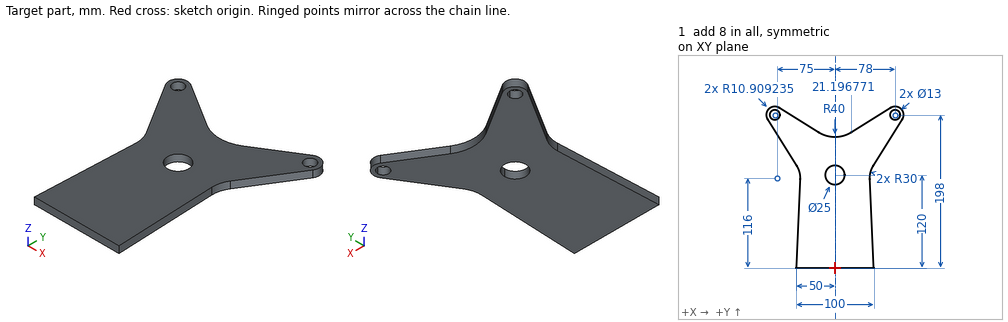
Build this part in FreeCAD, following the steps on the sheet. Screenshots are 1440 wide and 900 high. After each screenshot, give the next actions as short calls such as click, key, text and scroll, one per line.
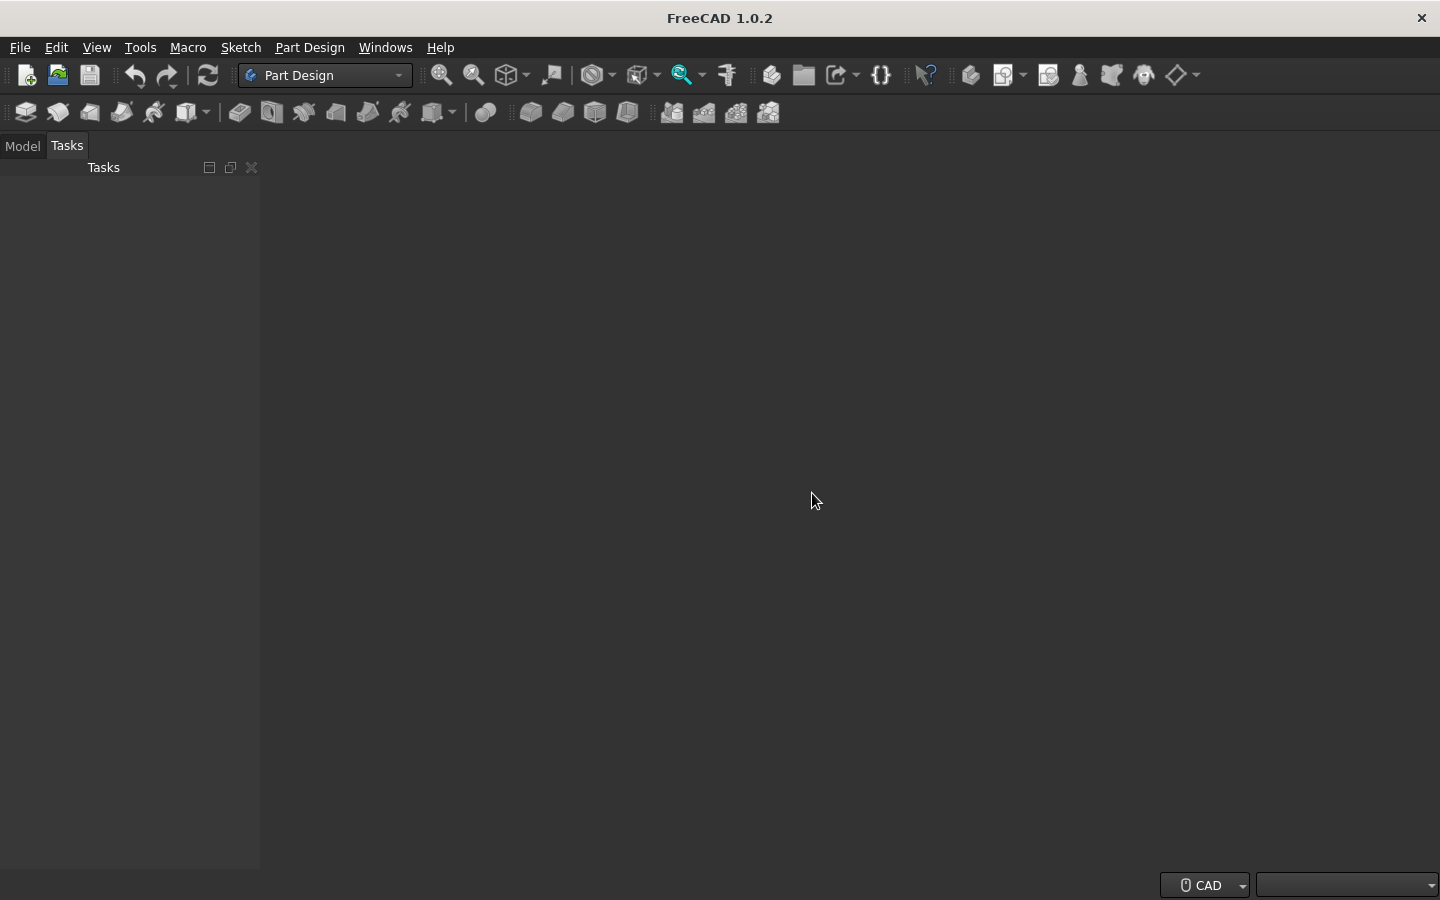
click(26, 76)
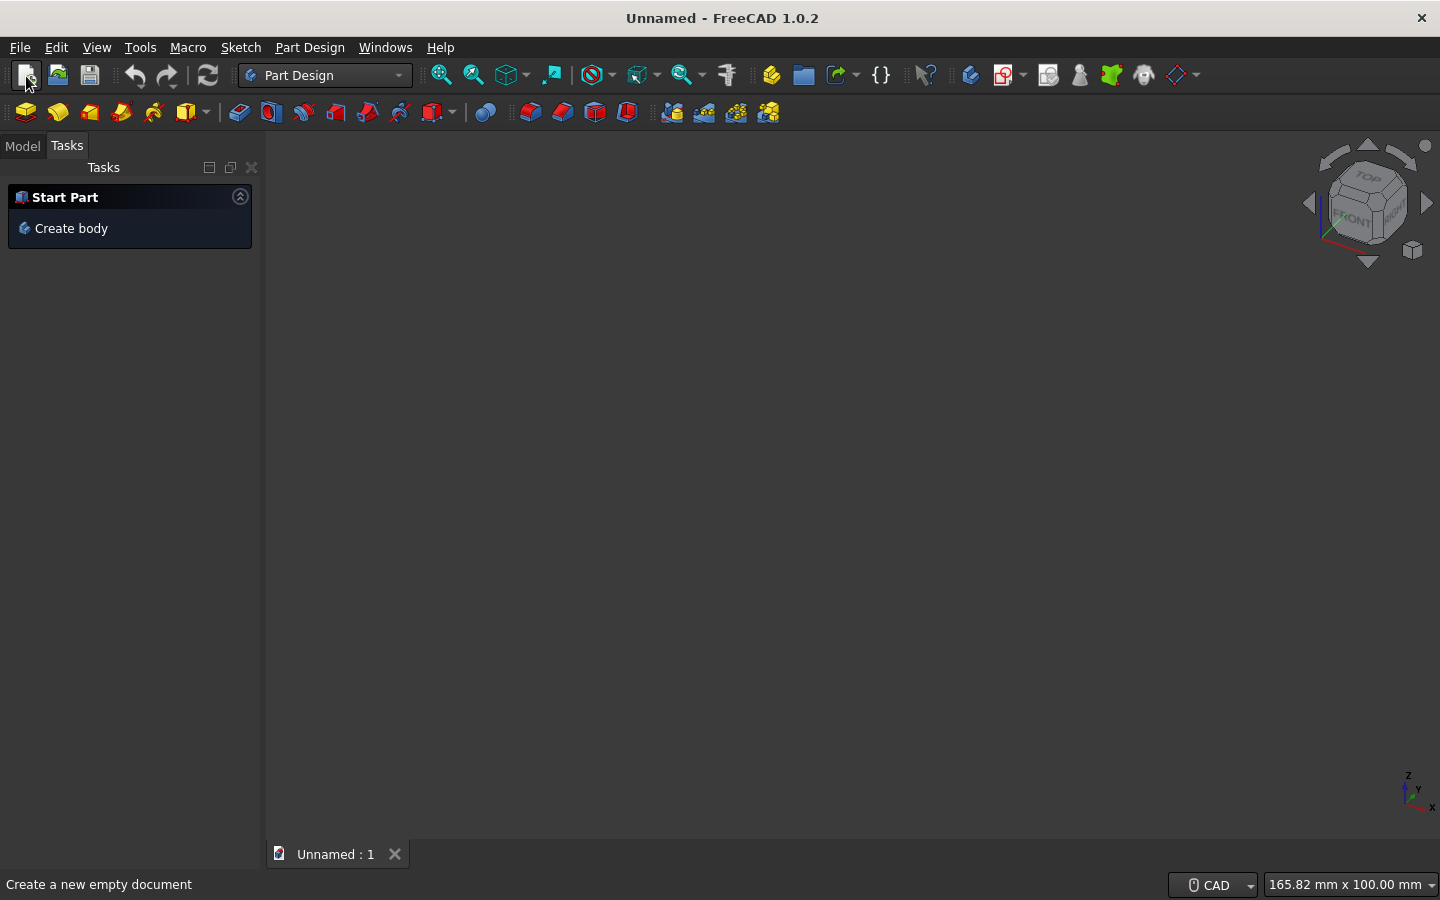
click(1004, 76)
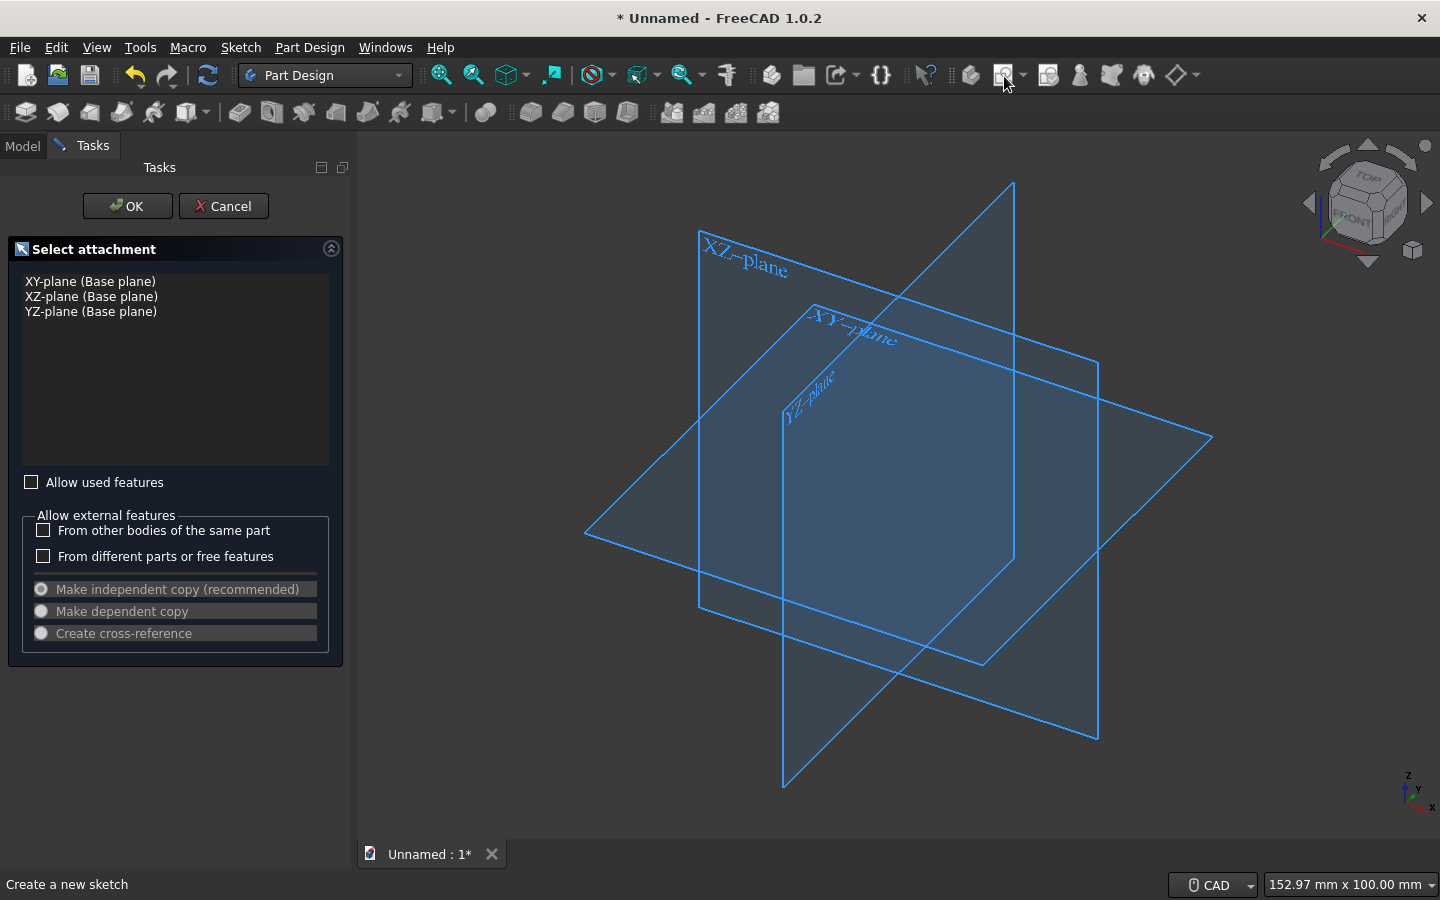
click(82, 282)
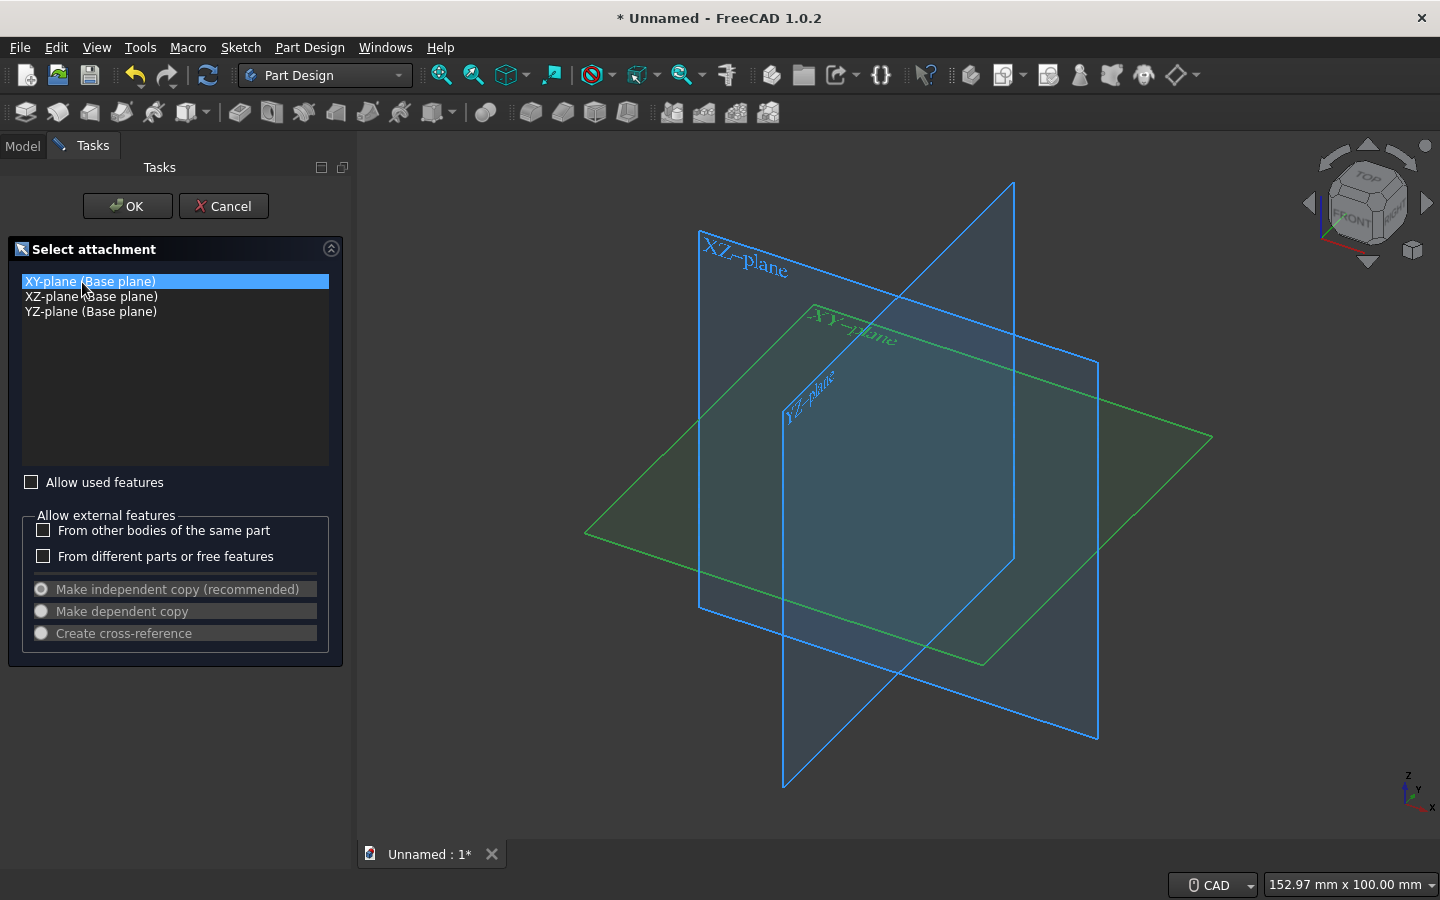
click(128, 206)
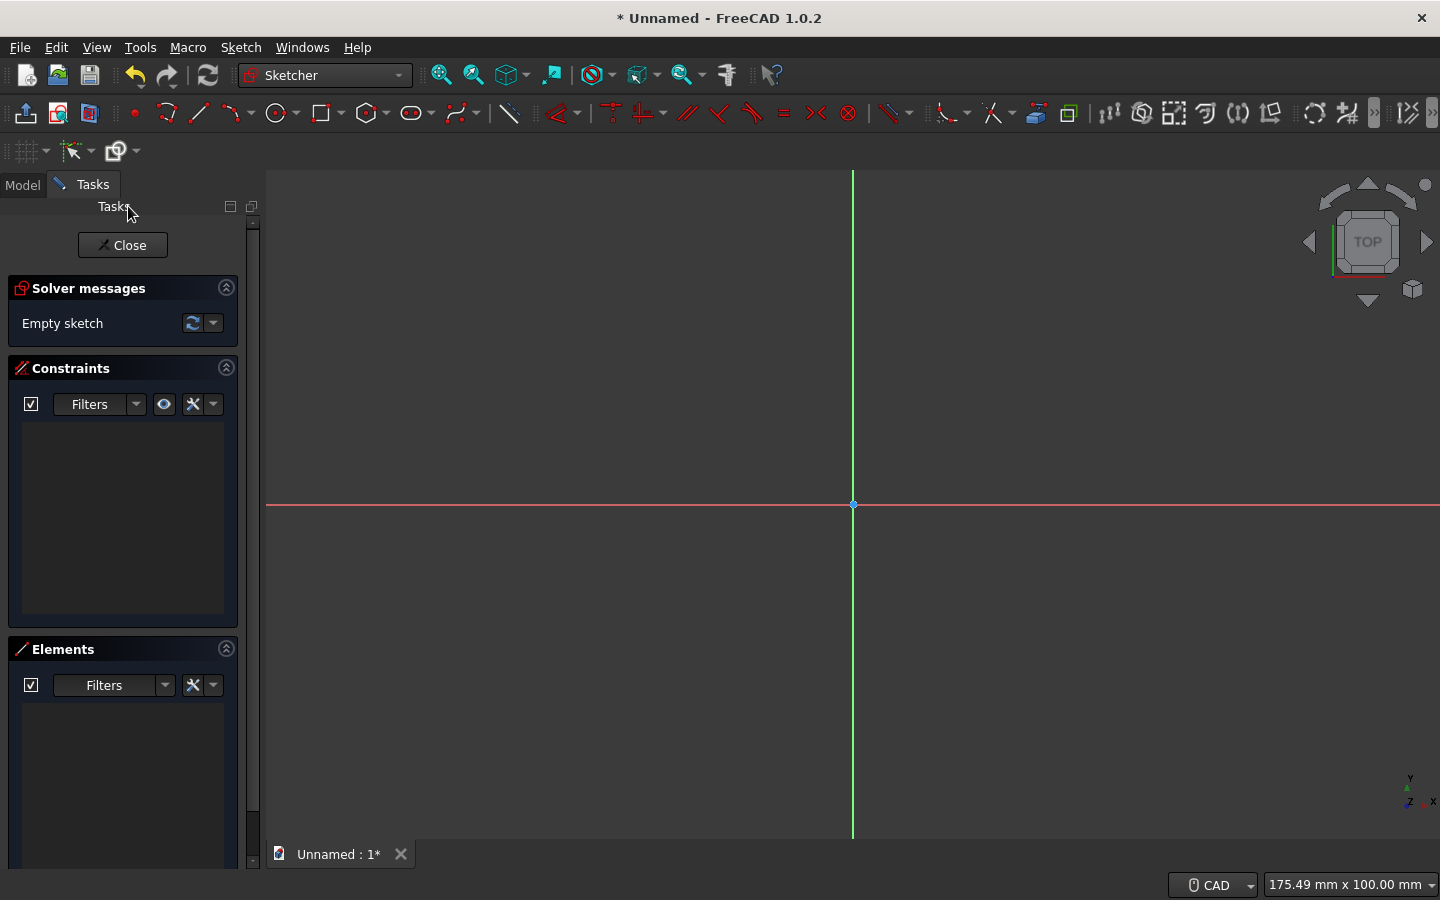
scroll(755, 803, down, 6)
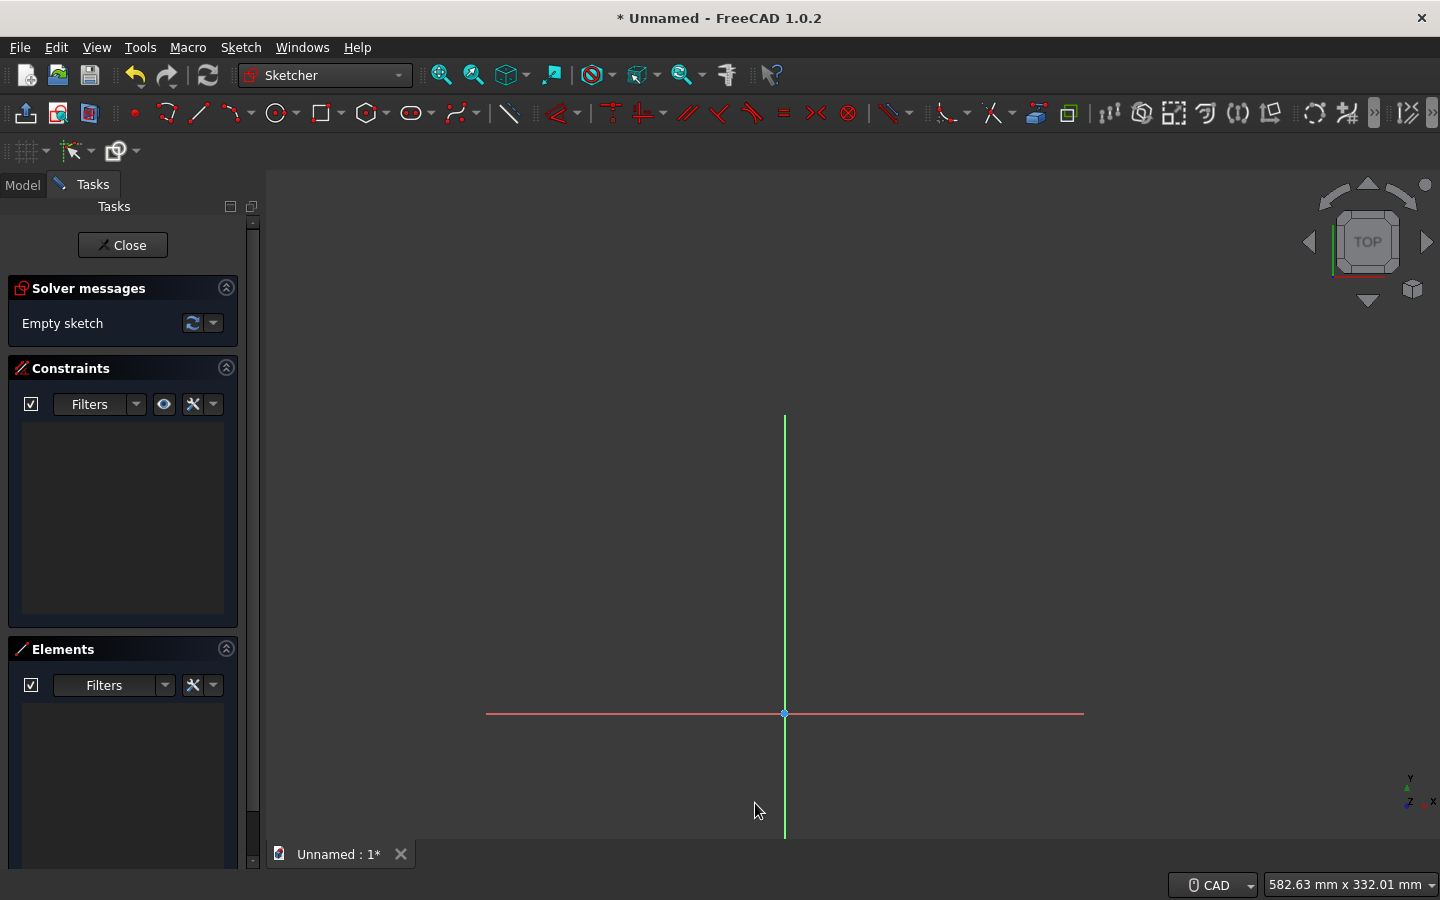
click(200, 114)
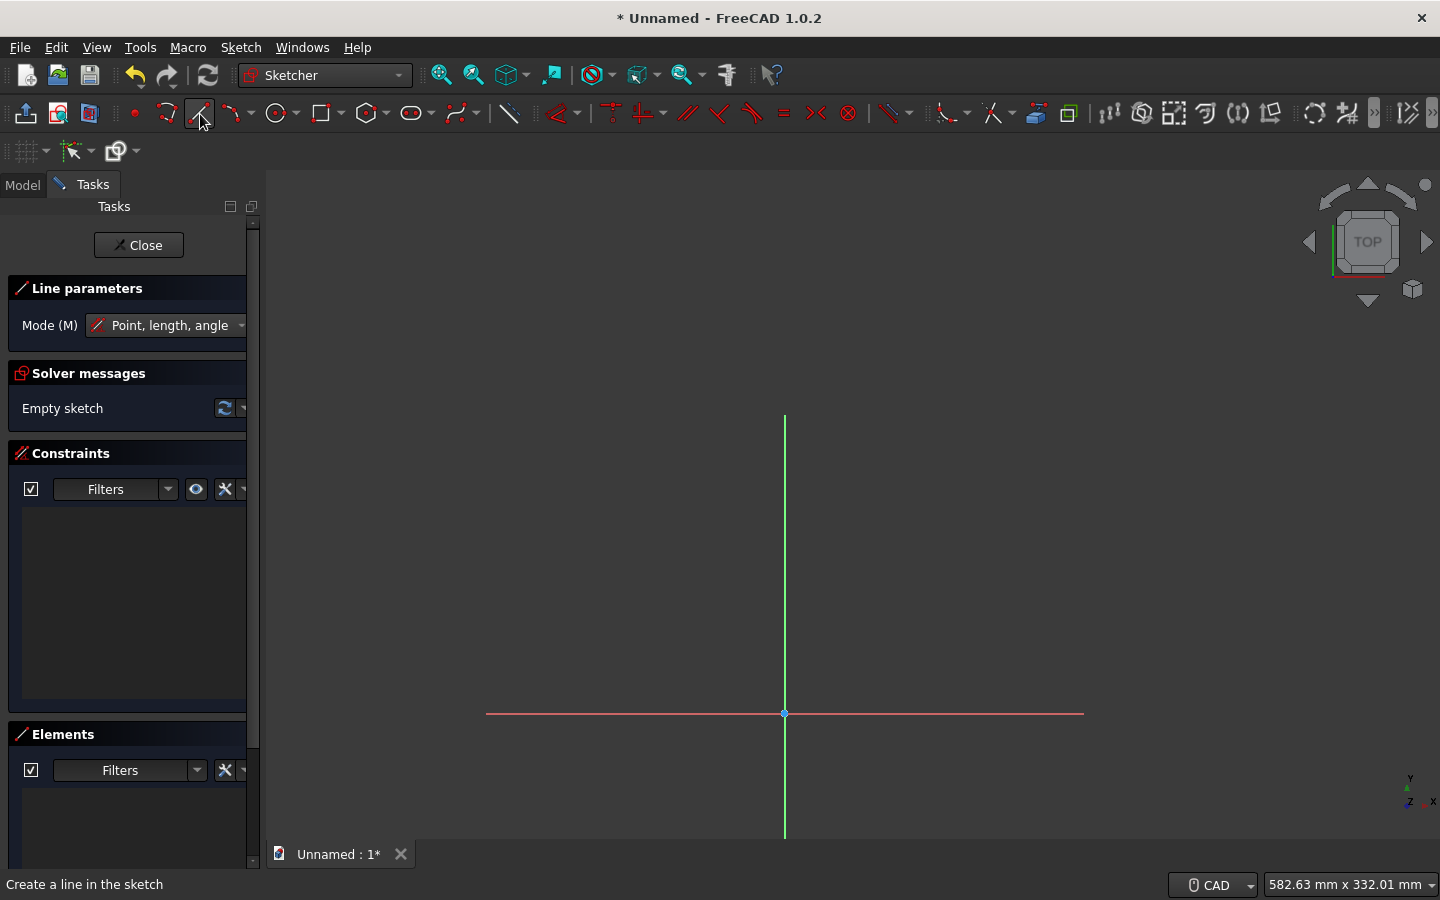
click(885, 448)
click(961, 326)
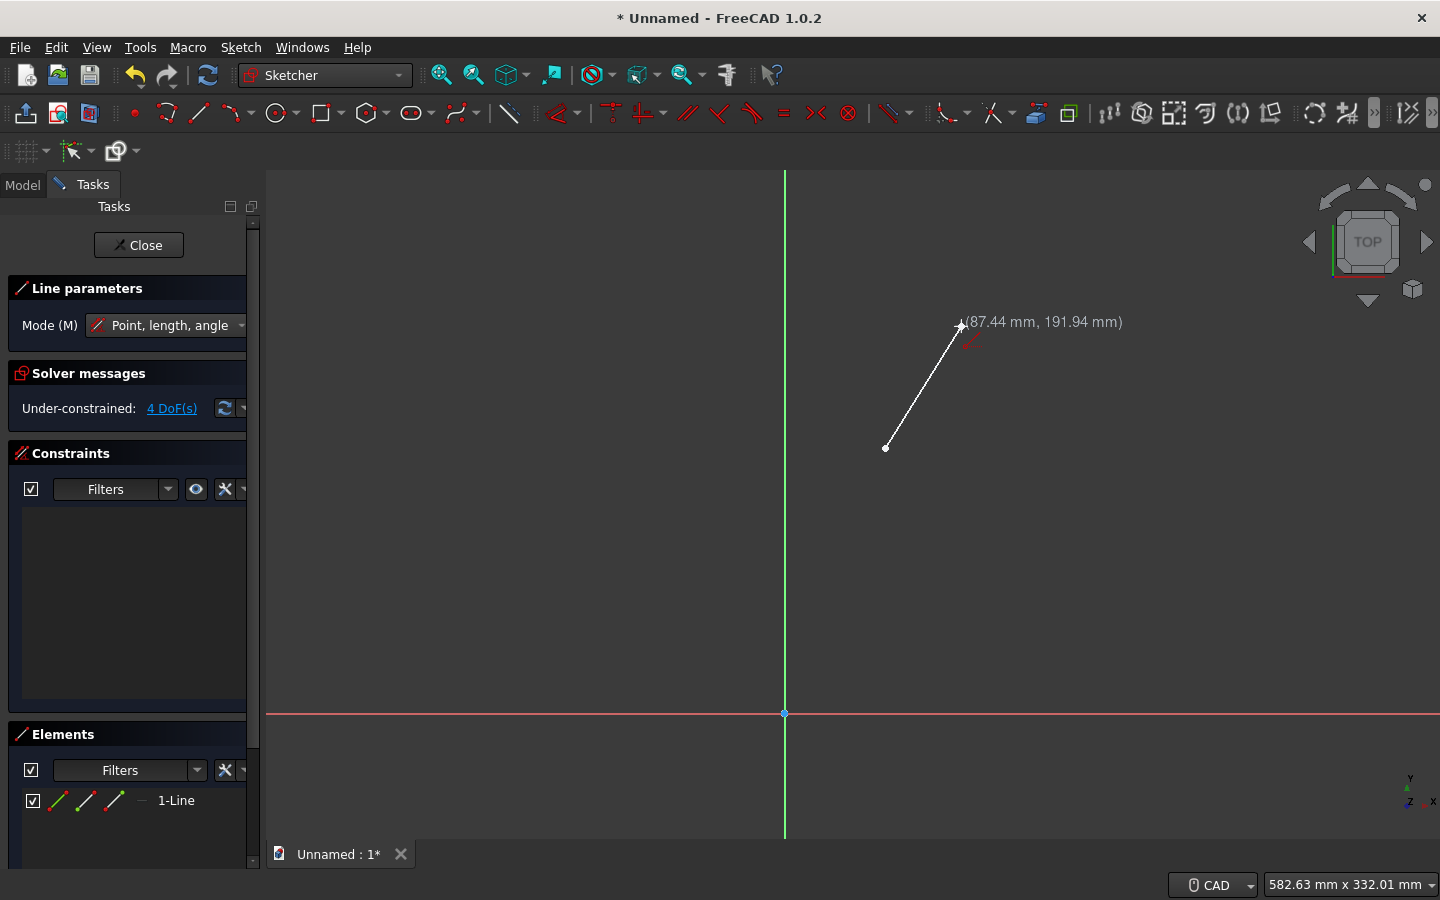
click(930, 296)
click(828, 360)